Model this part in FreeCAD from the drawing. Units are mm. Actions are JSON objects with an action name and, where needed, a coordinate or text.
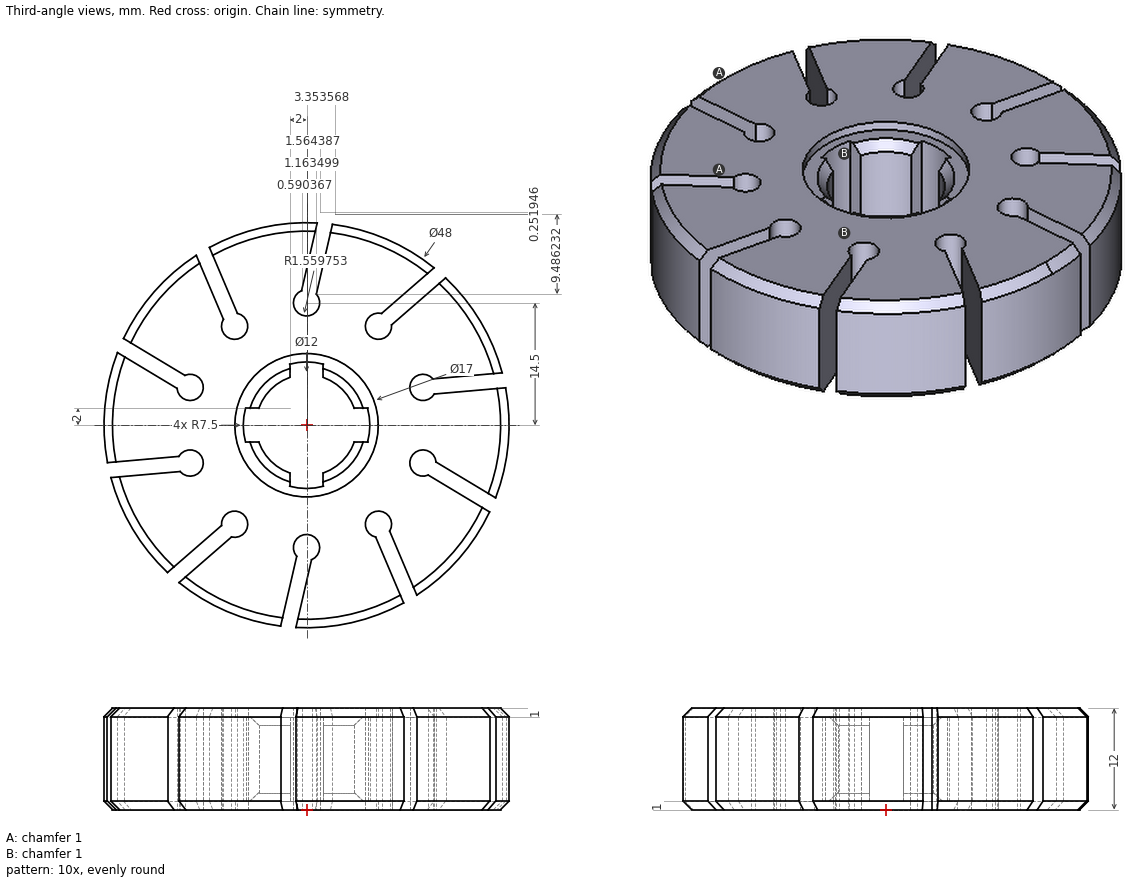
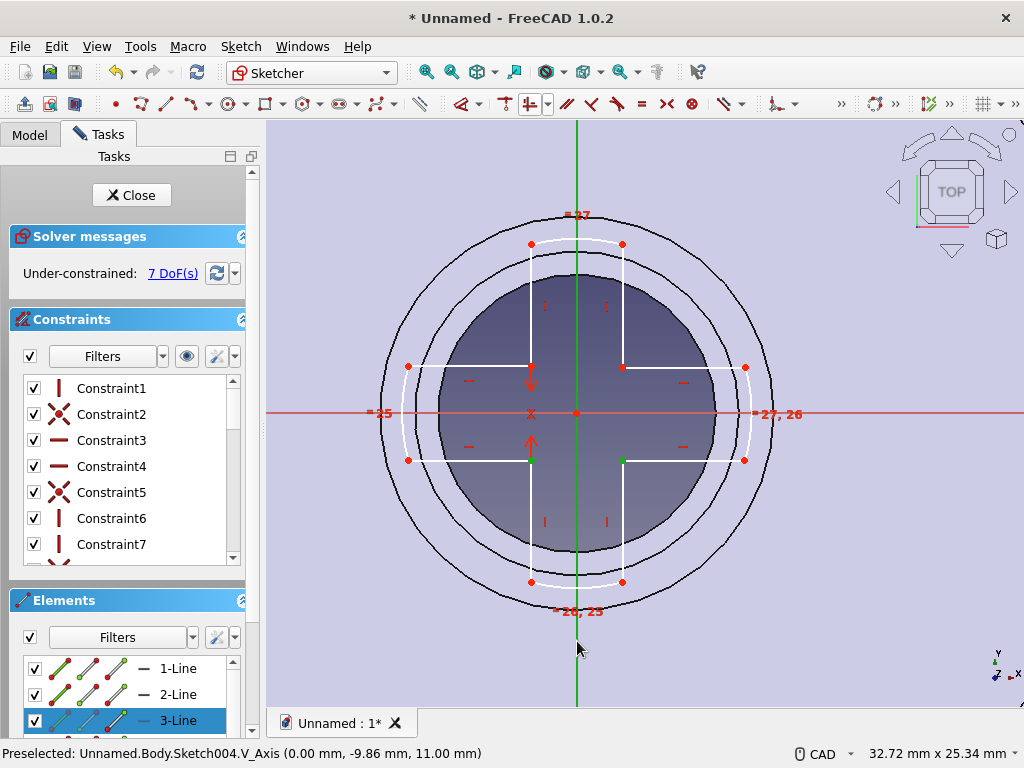
{"action": "left_click", "coordinate": [667, 104]}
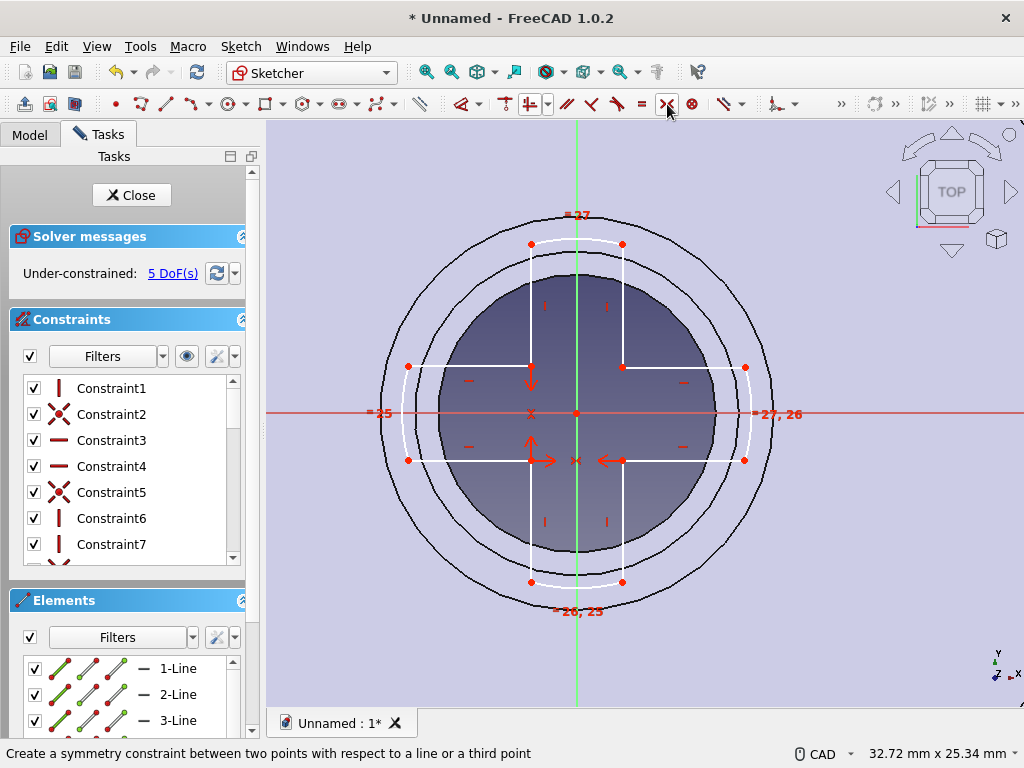
{"action": "left_click", "coordinate": [531, 366]}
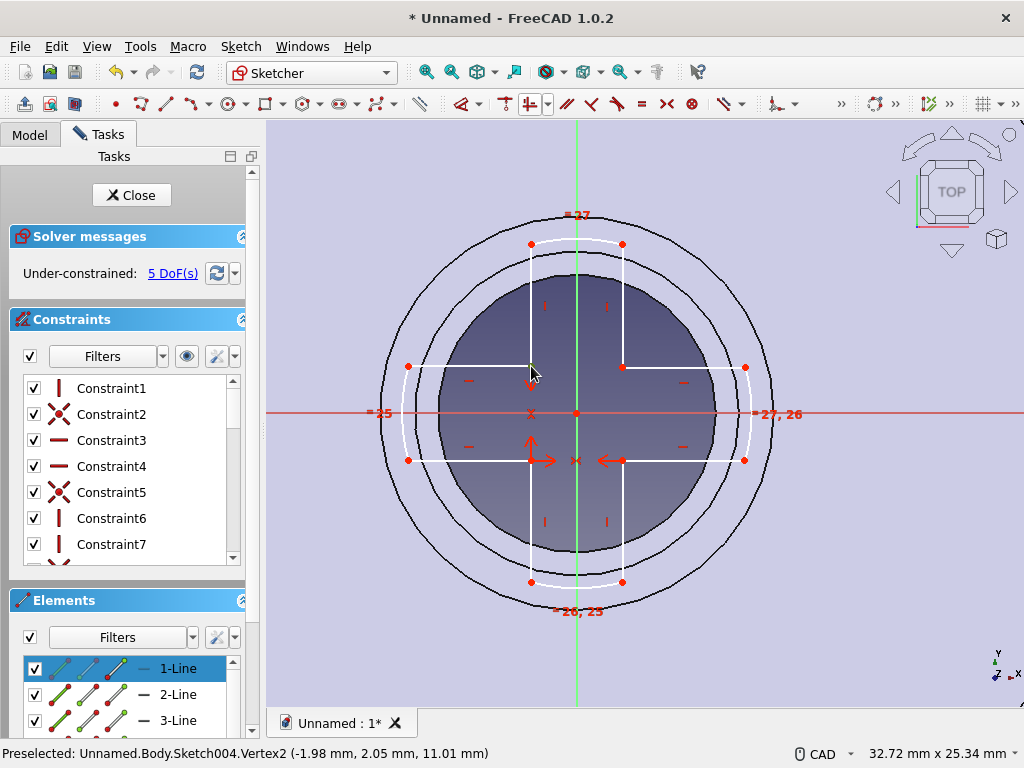
{"action": "left_click", "coordinate": [623, 368]}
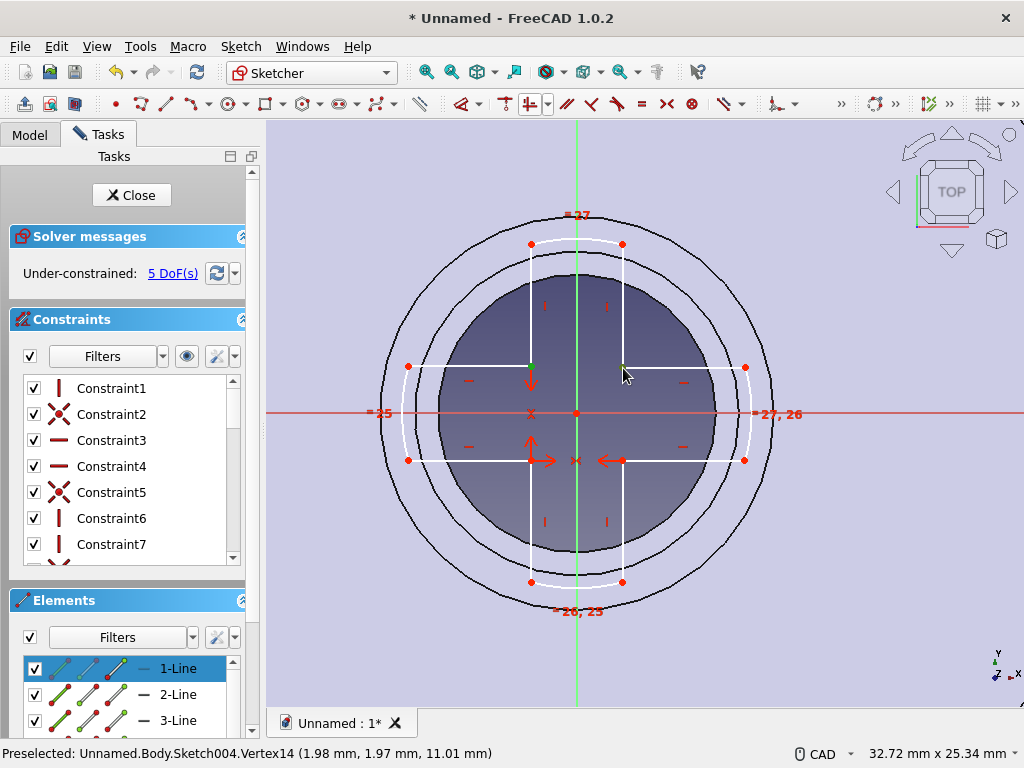
{"action": "left_click", "coordinate": [577, 641]}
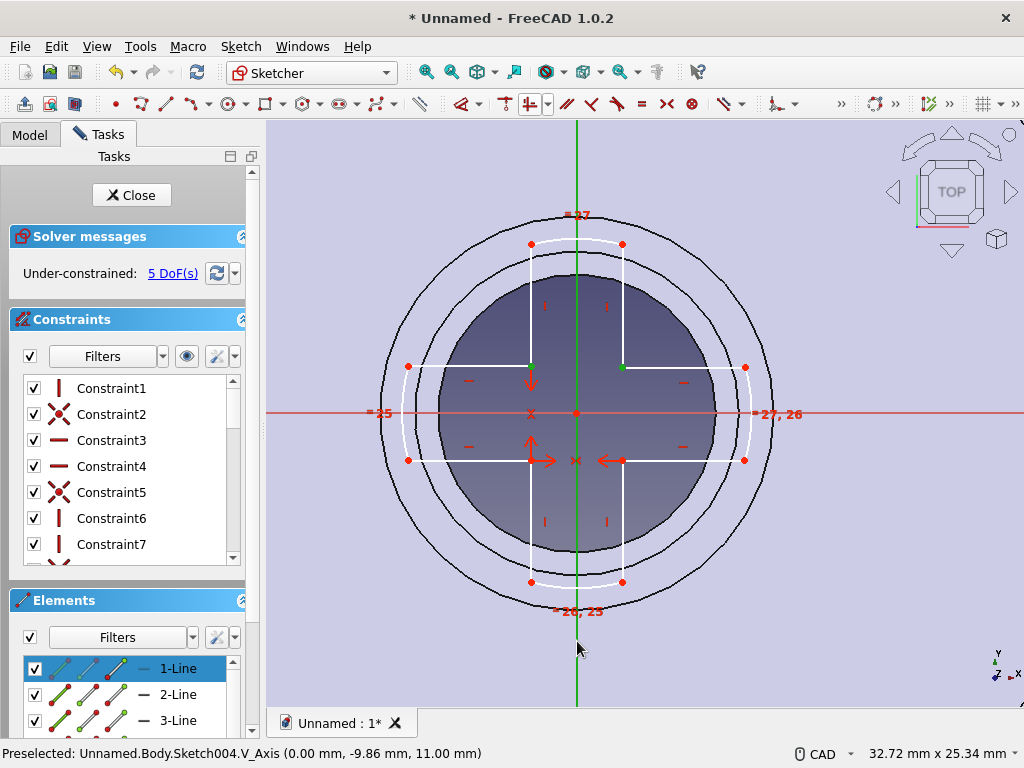
{"action": "left_click", "coordinate": [667, 104]}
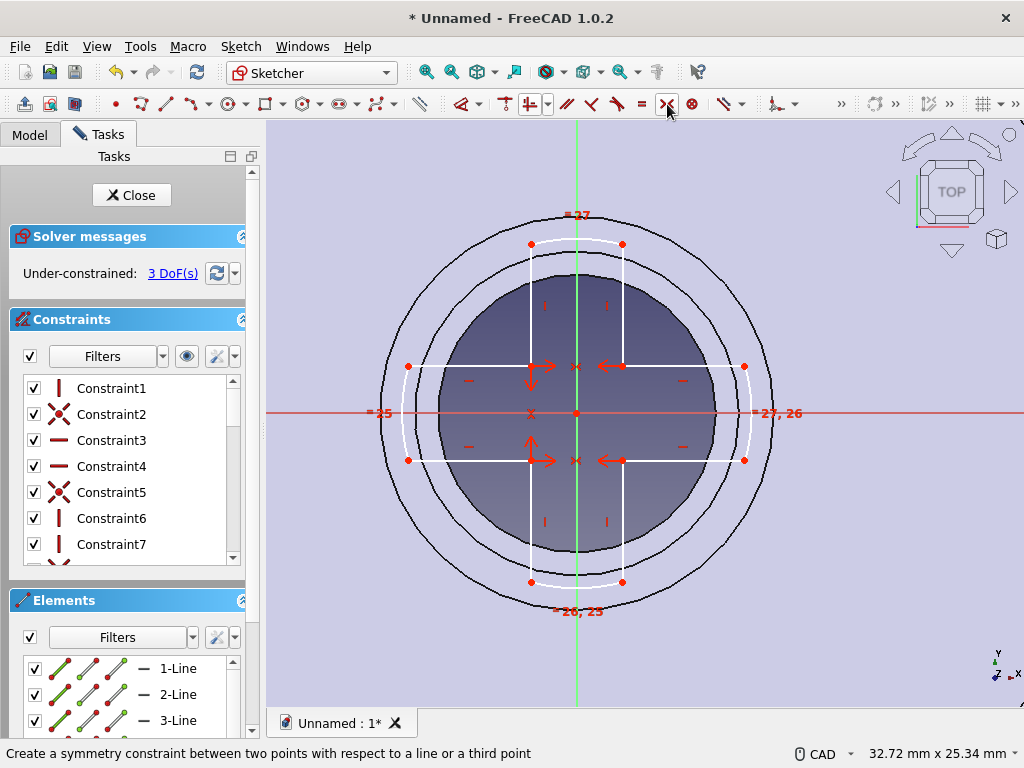
{"action": "left_click", "coordinate": [460, 104]}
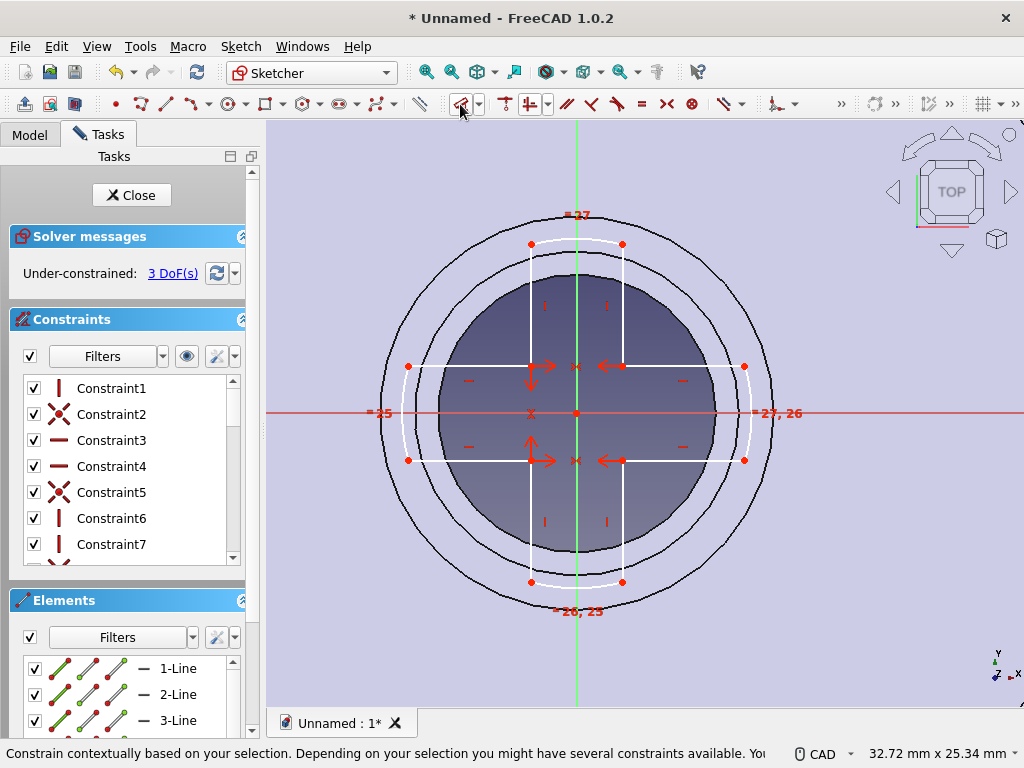
{"action": "left_click", "coordinate": [403, 394]}
{"action": "left_click", "coordinate": [371, 390]}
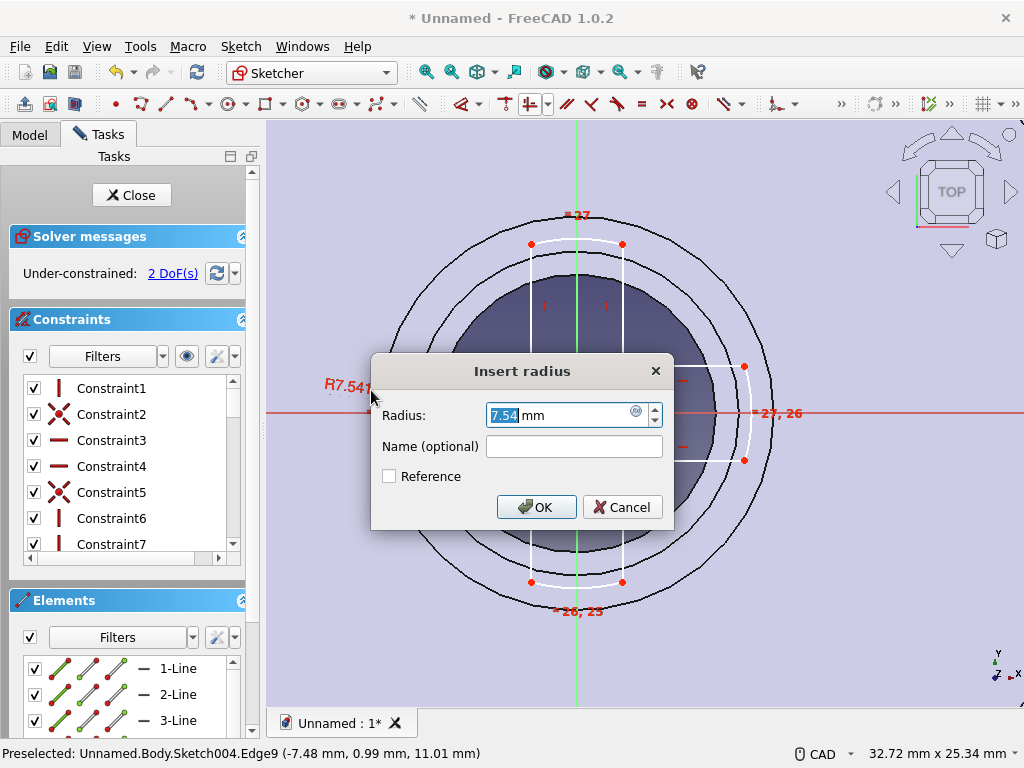
{"action": "type", "text": "7.5"}
{"action": "key", "text": "Return"}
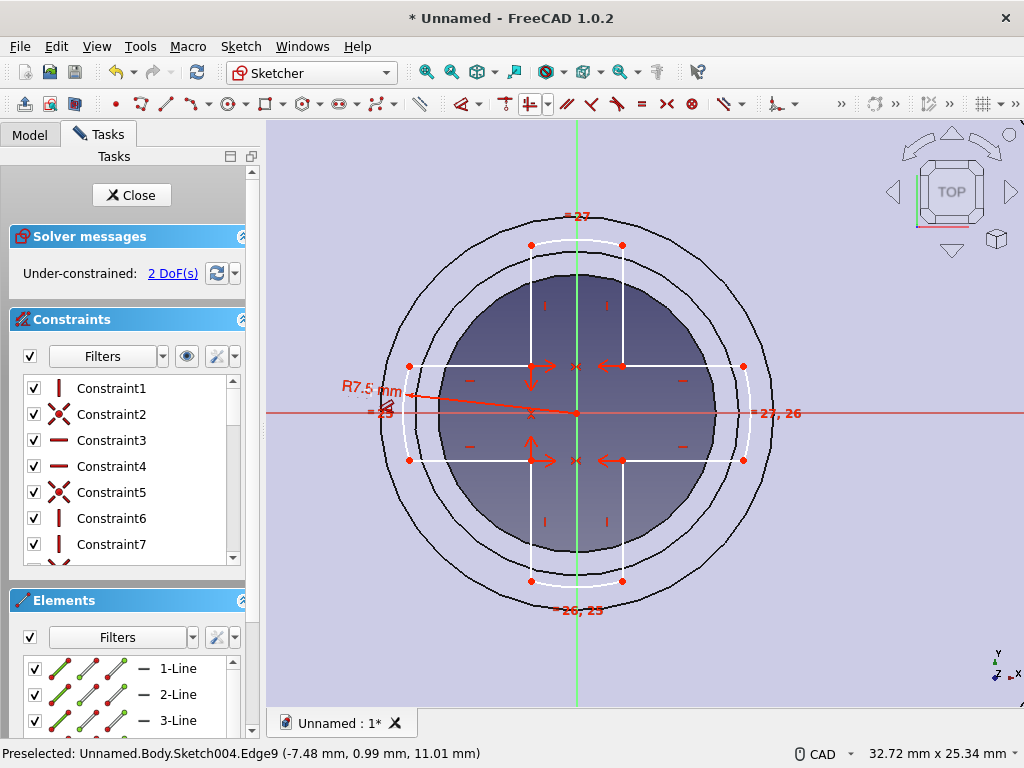
{"action": "left_click", "coordinate": [531, 246]}
{"action": "left_click", "coordinate": [554, 212]}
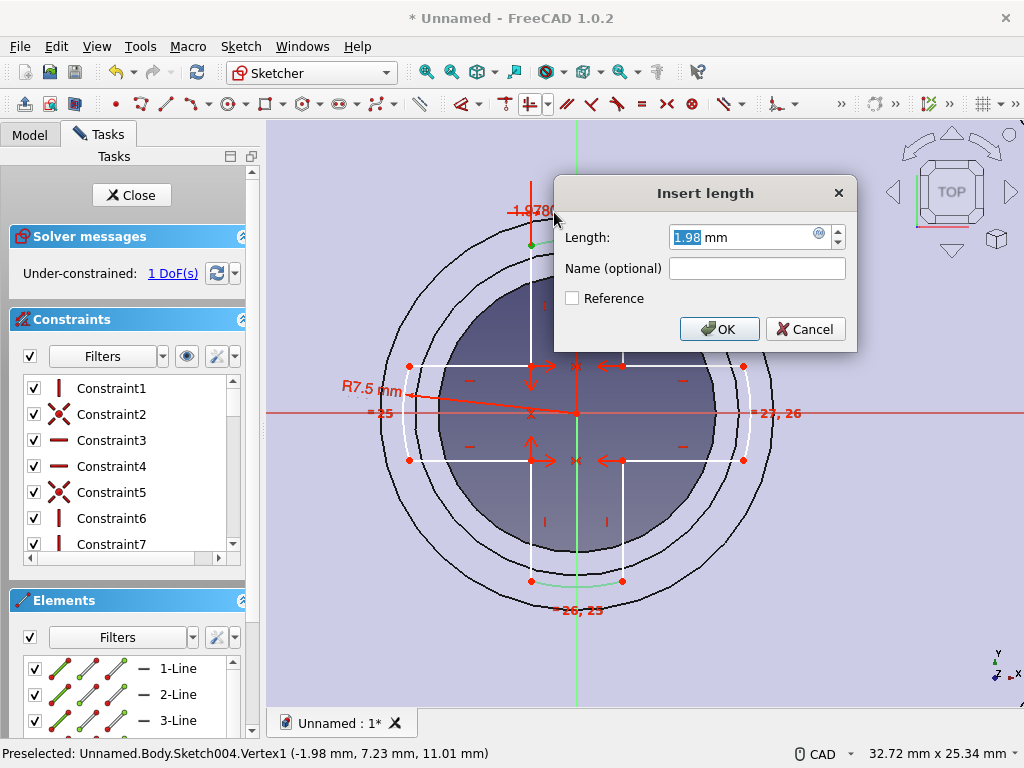
{"action": "type", "text": "2"}
{"action": "key", "text": "Return"}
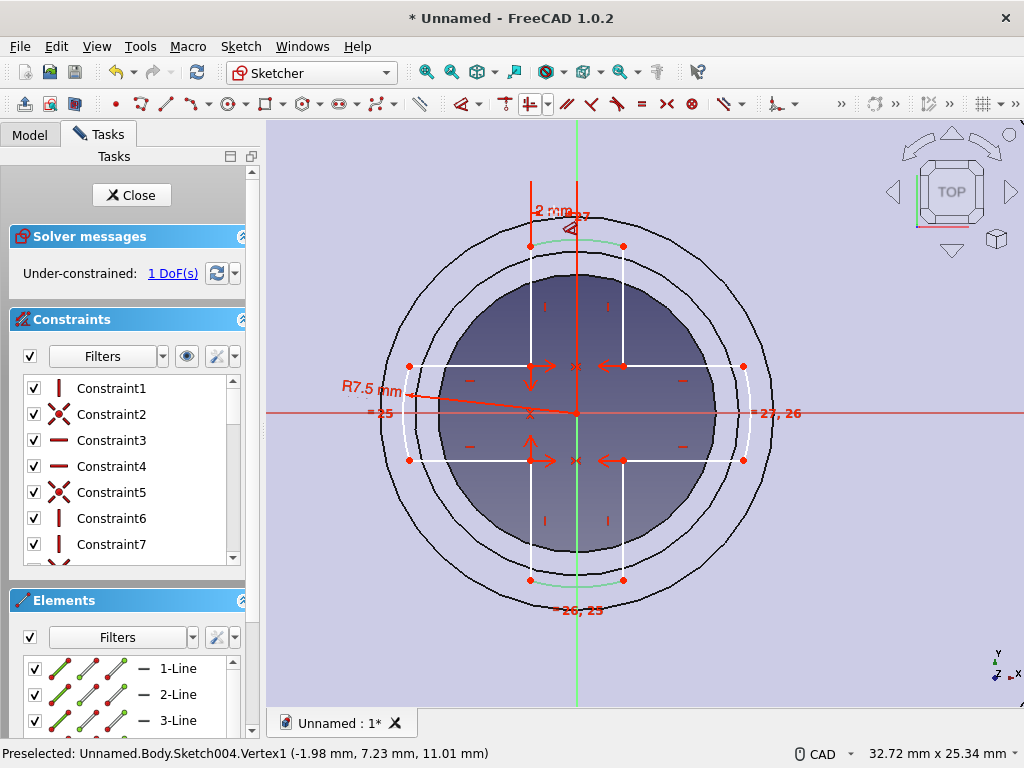
{"action": "left_click", "coordinate": [531, 366]}
{"action": "left_click", "coordinate": [497, 390]}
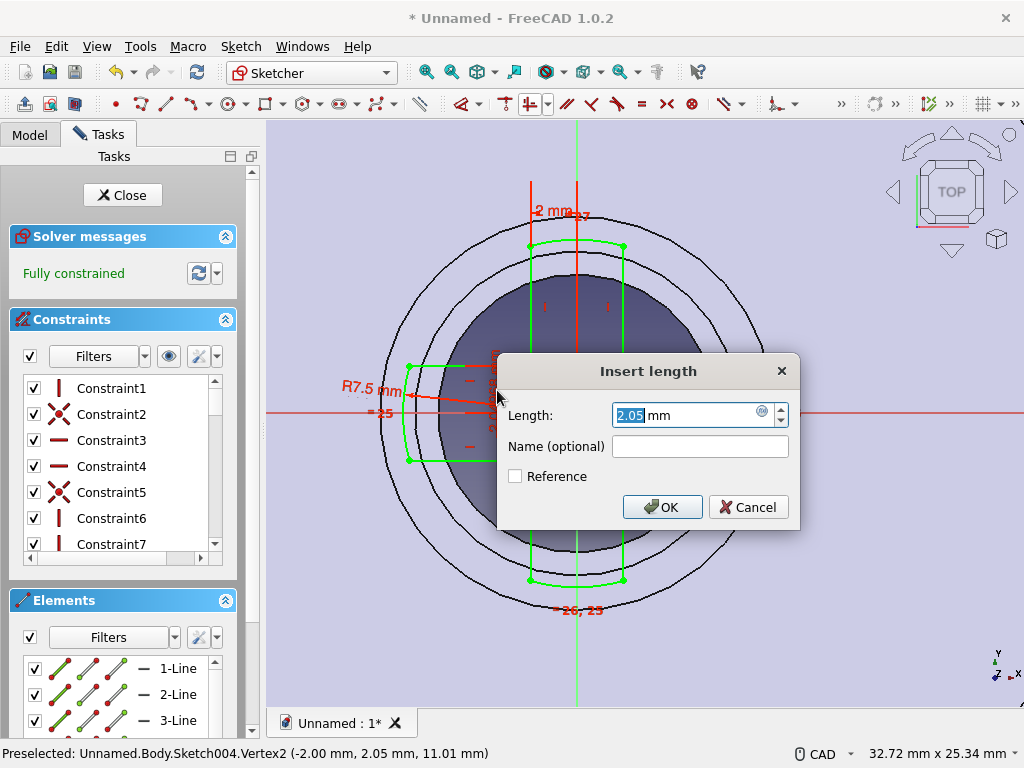
{"action": "type", "text": "2"}
{"action": "key", "text": "Return"}
{"action": "key", "text": "Escape"}